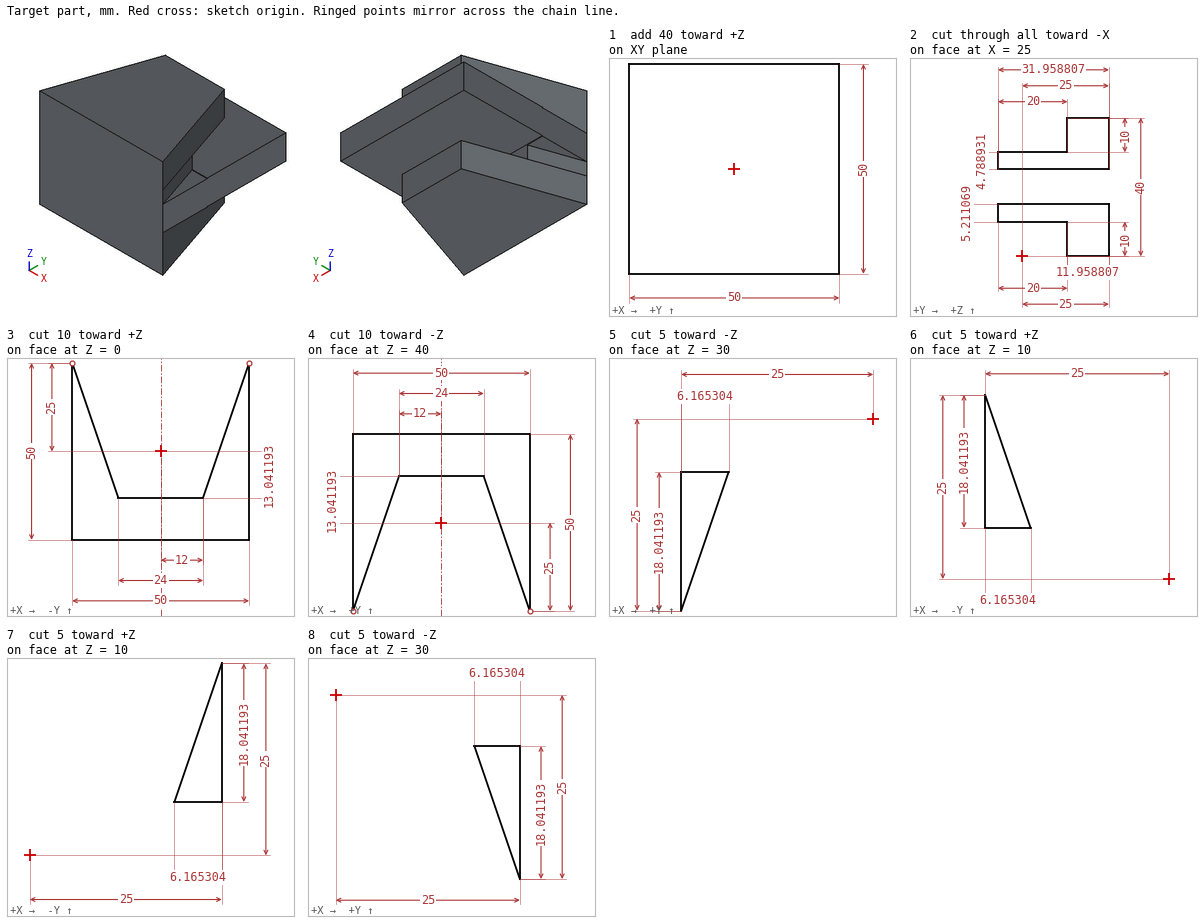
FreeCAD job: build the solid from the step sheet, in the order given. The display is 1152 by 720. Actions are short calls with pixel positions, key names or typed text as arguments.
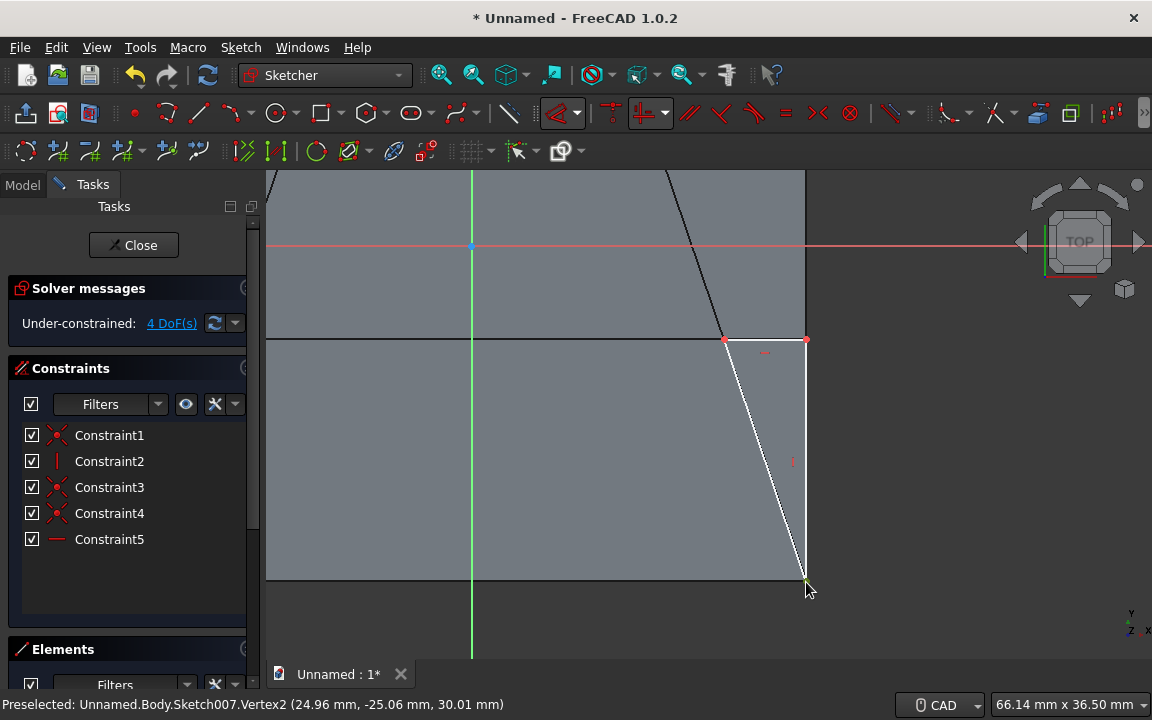
key(l)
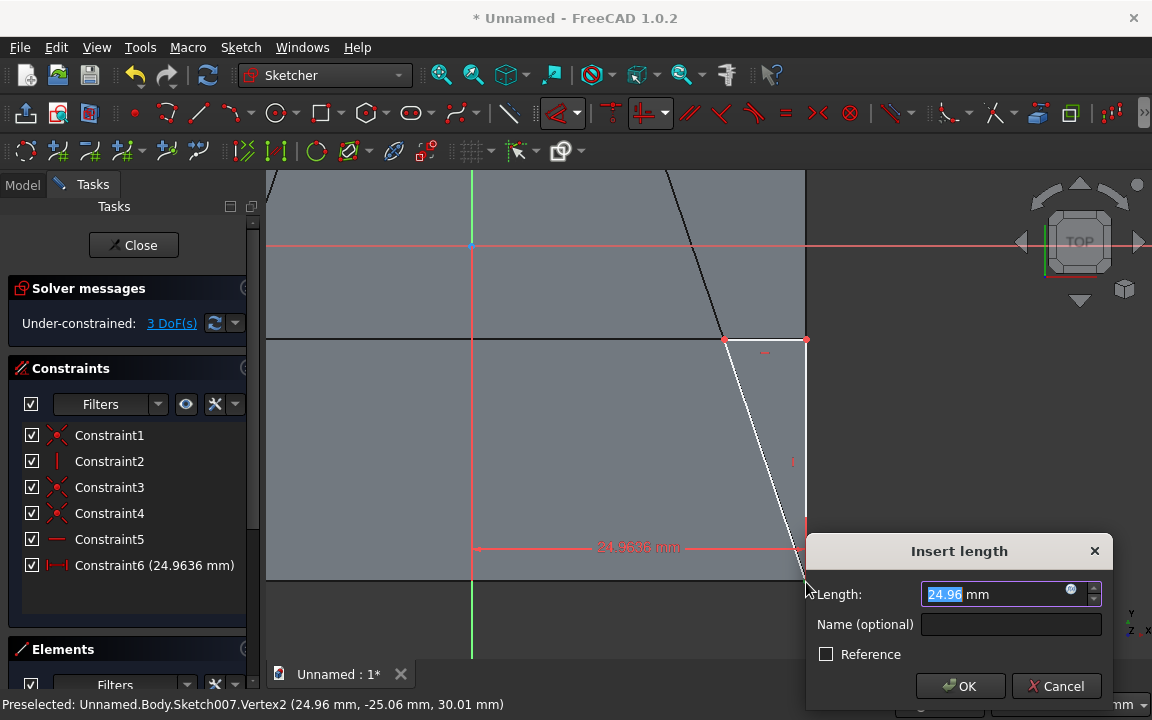
text(25)
key(Return)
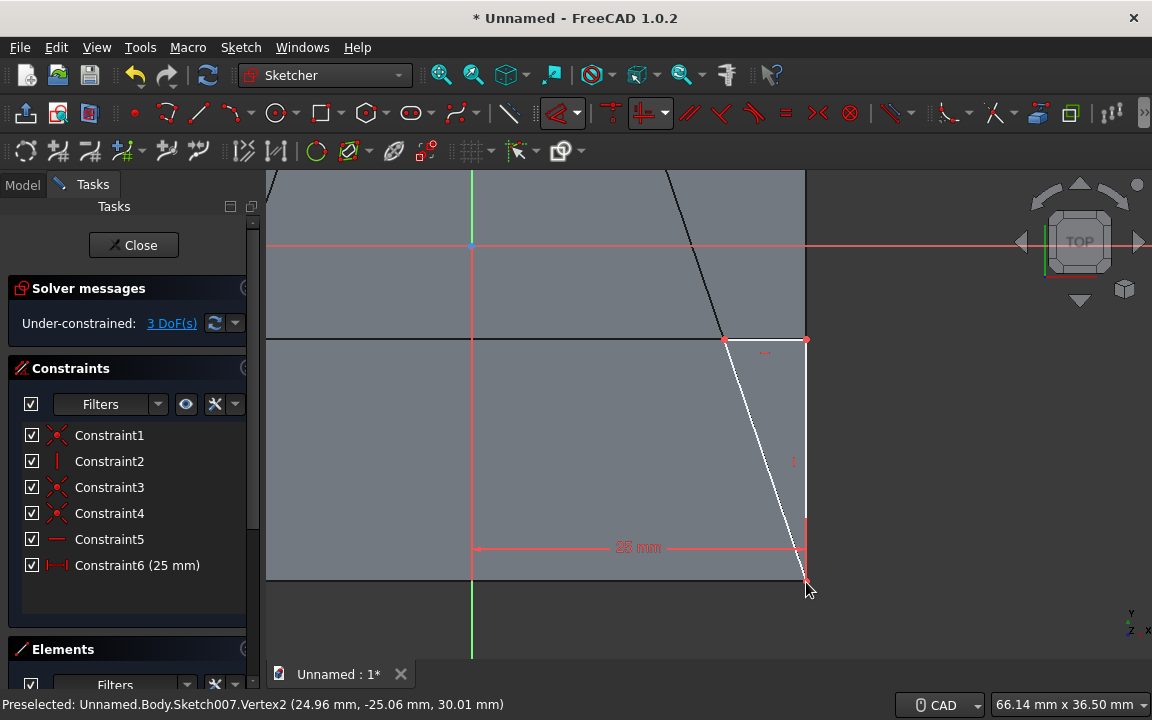
click(806, 582)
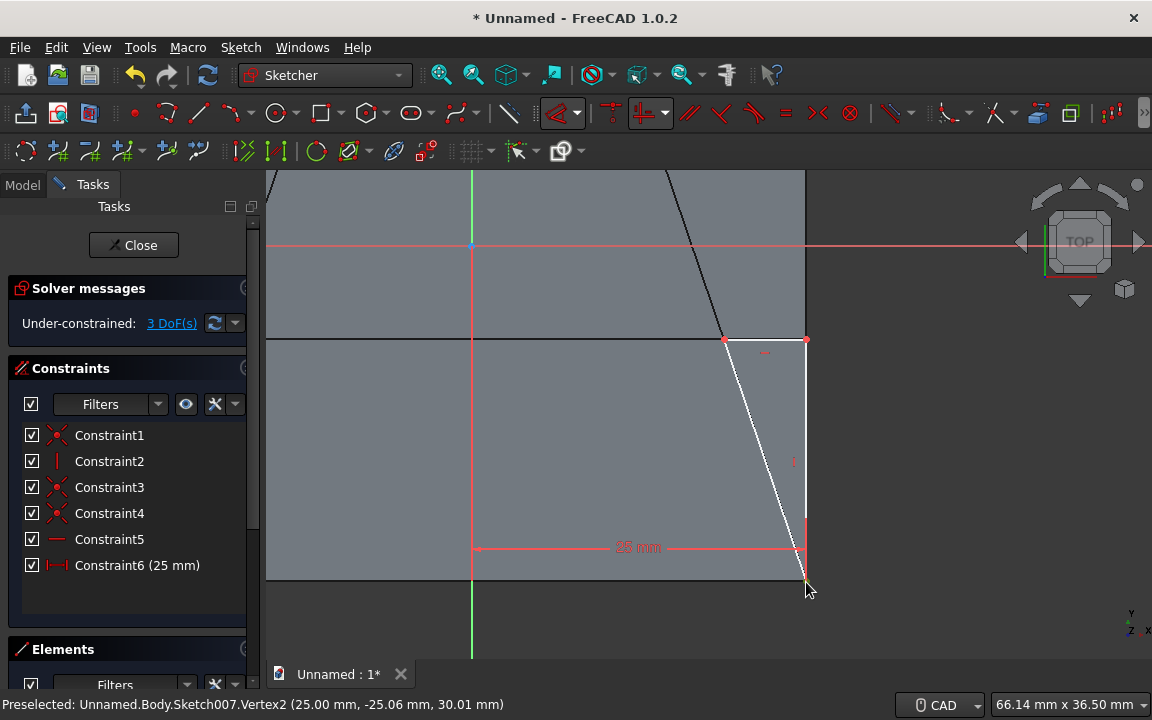
key(i)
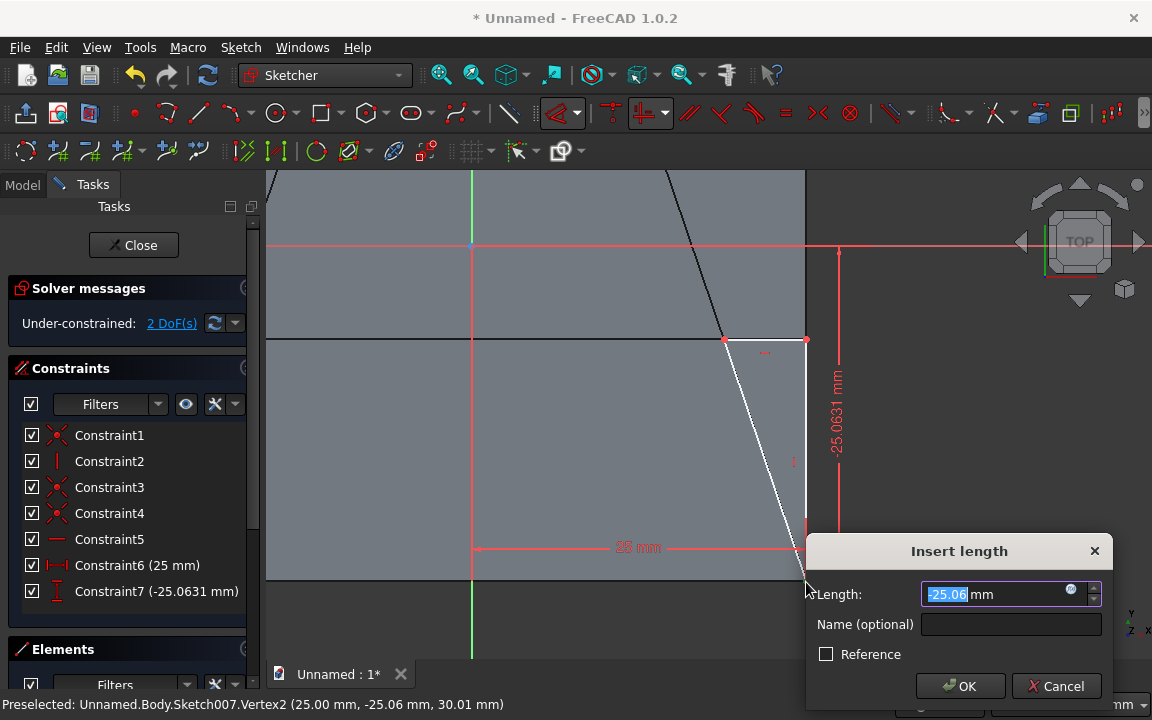
text(-25)
key(Return)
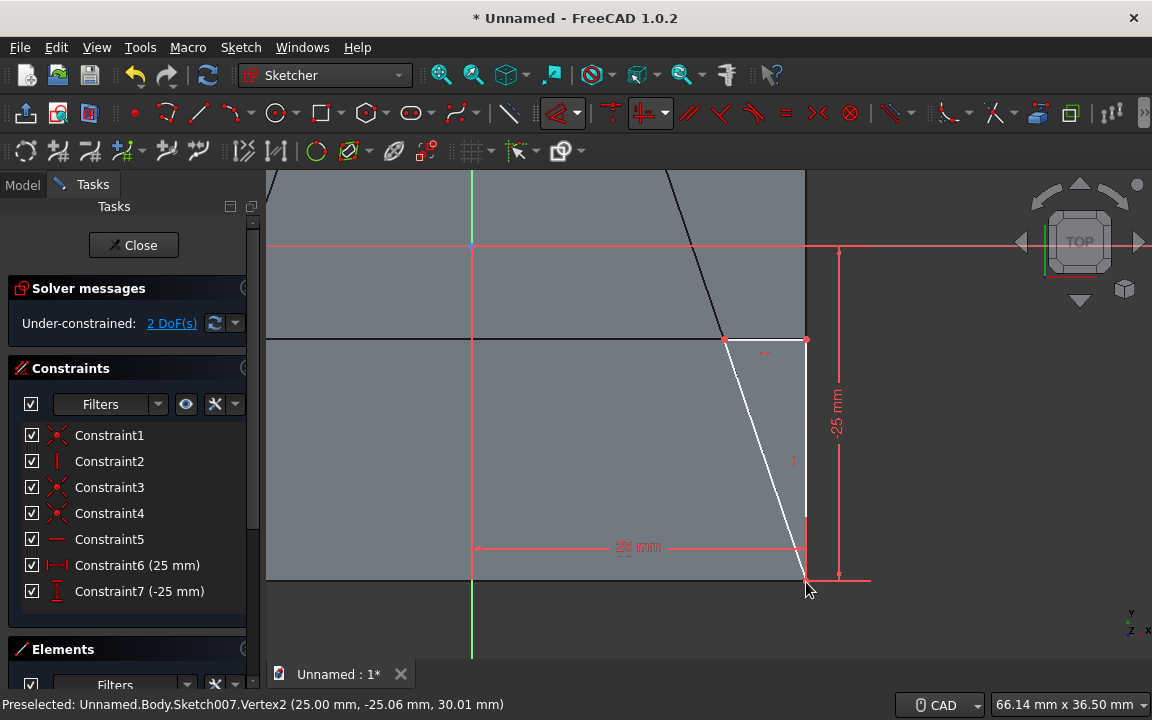
click(782, 340)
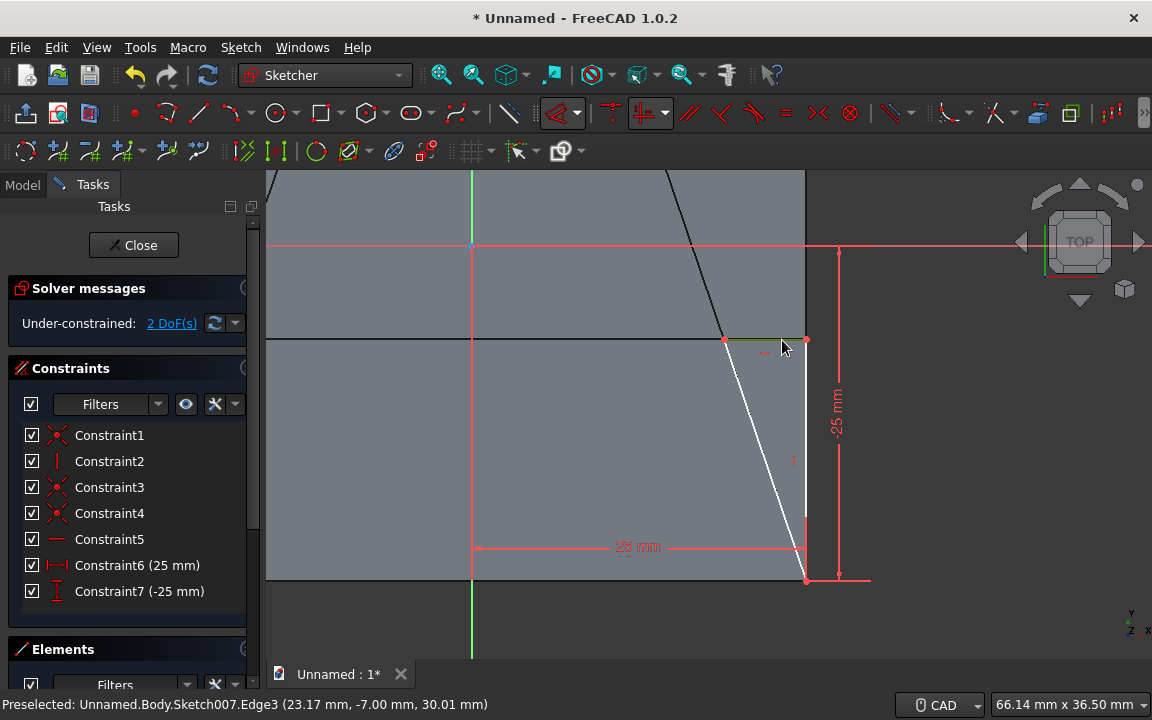
key(l)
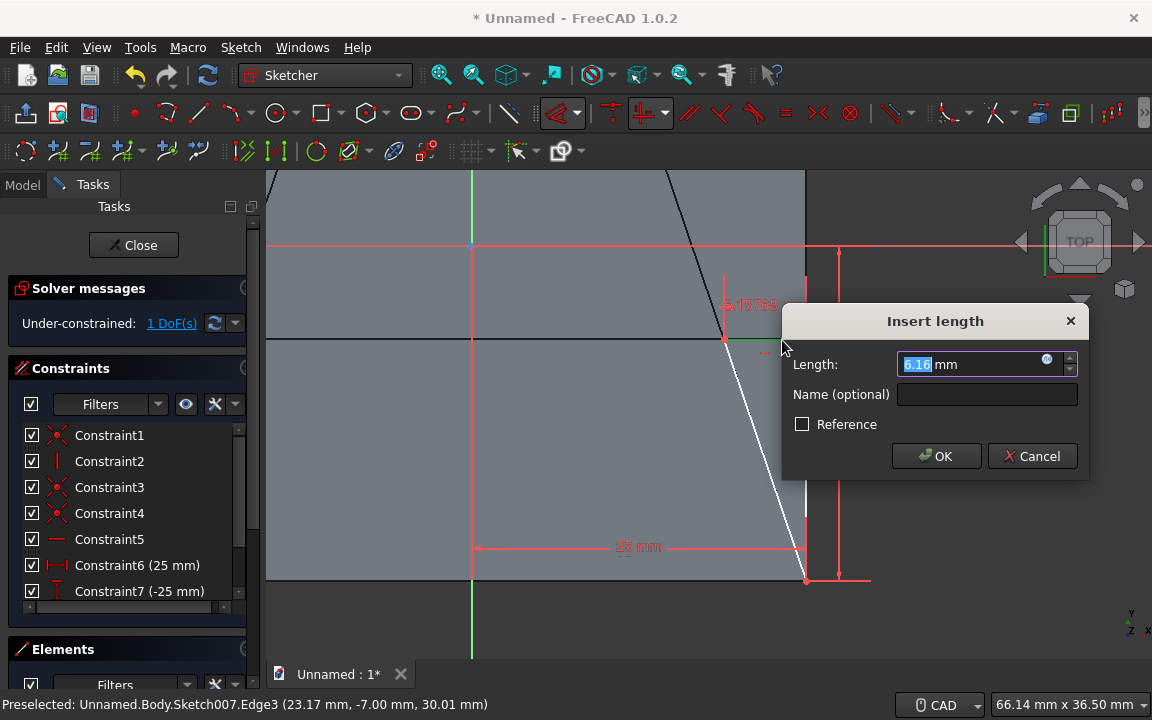
text(6.165304)
key(Return)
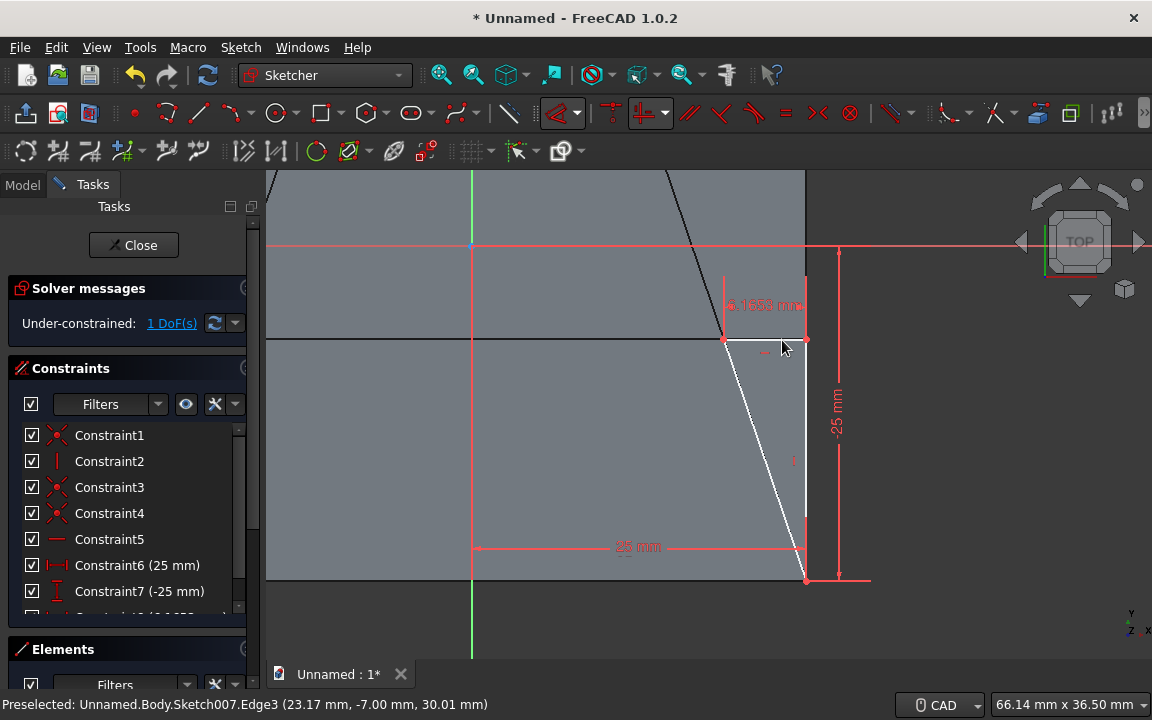
click(806, 509)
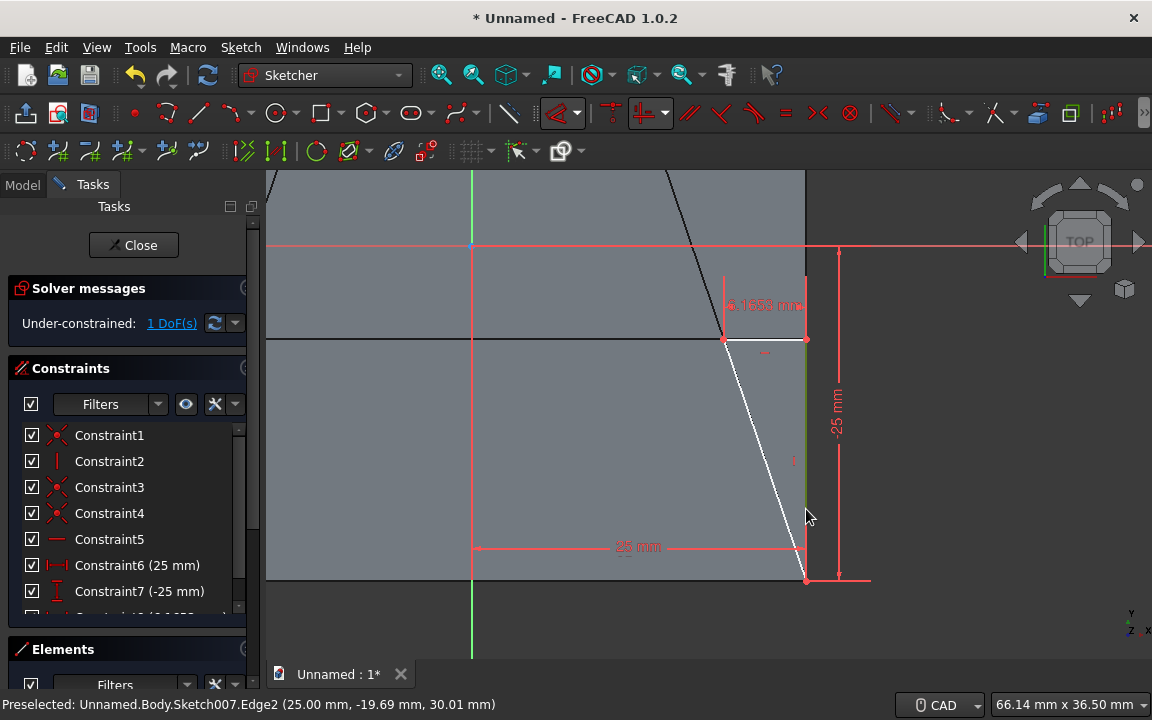
key(i)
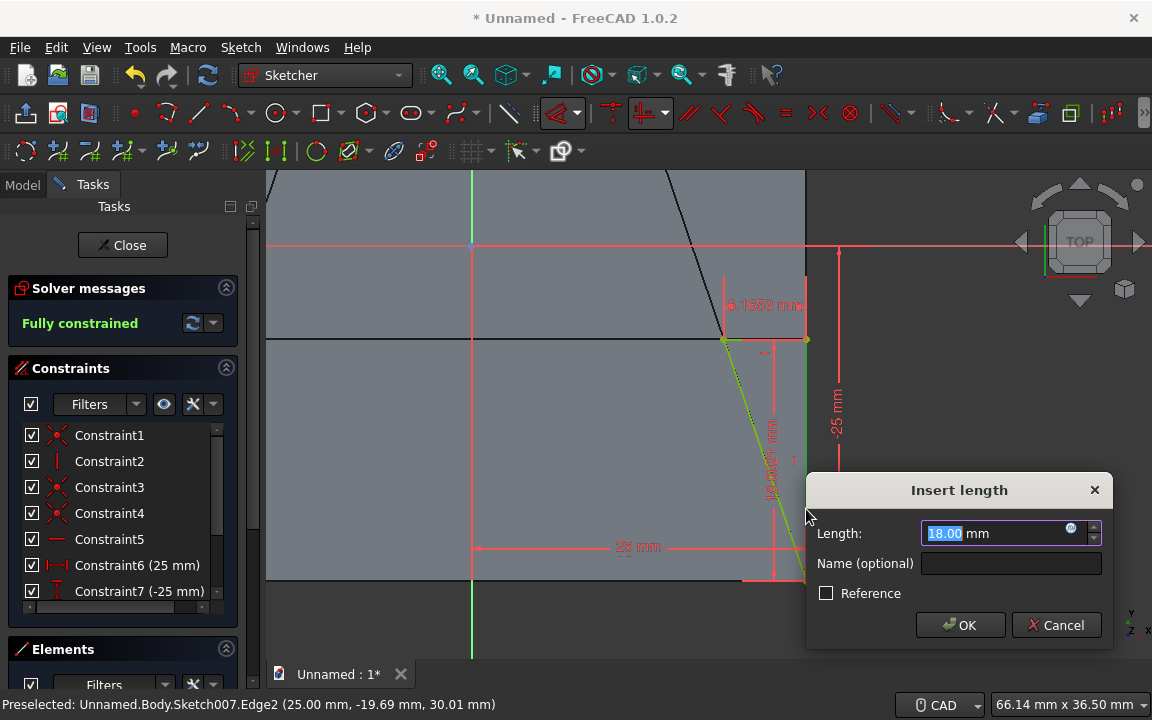
text(18.041193)
key(Return)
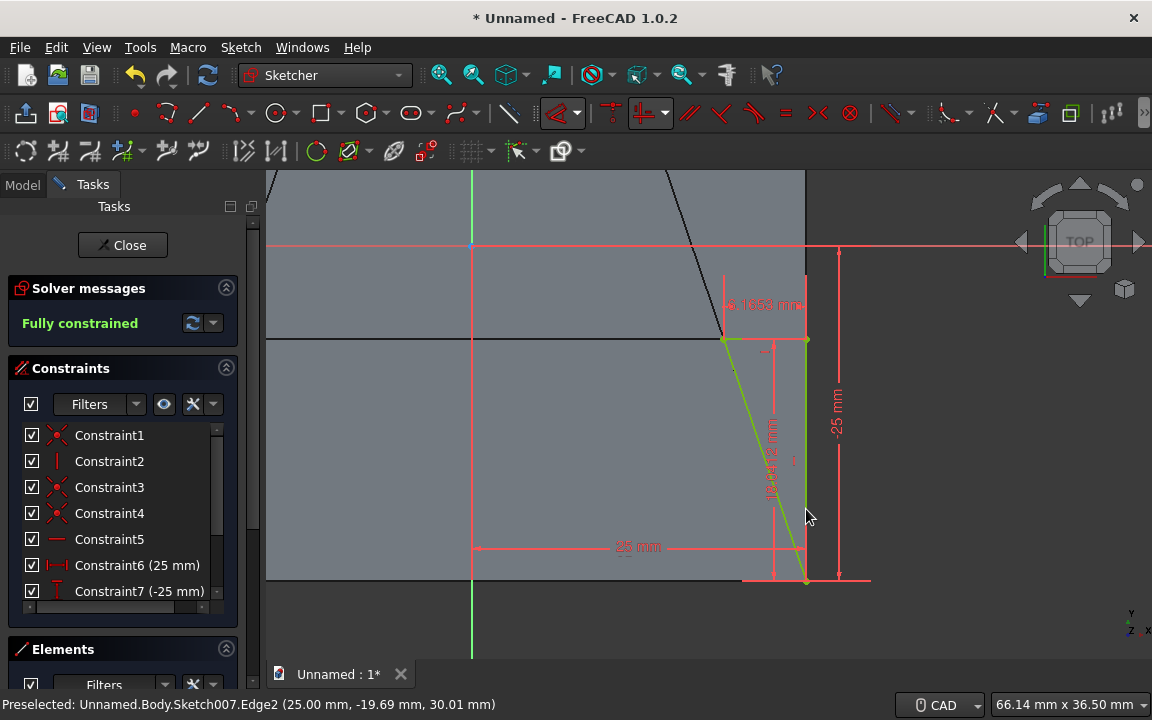
click(123, 245)